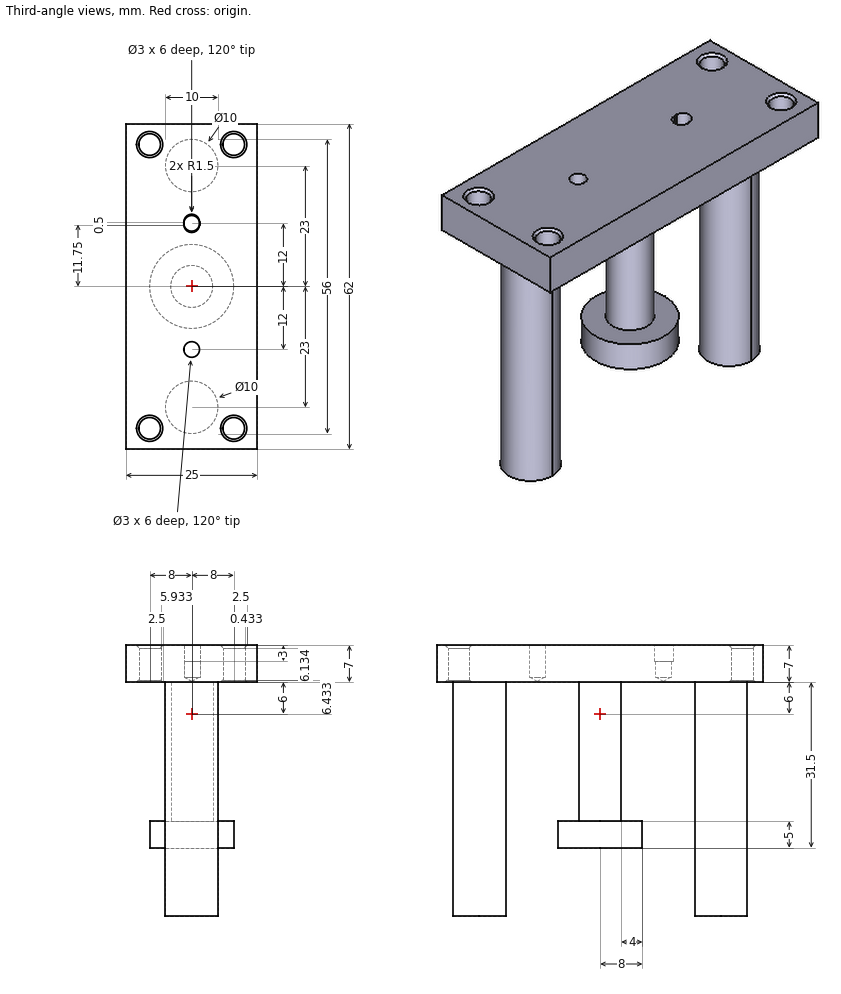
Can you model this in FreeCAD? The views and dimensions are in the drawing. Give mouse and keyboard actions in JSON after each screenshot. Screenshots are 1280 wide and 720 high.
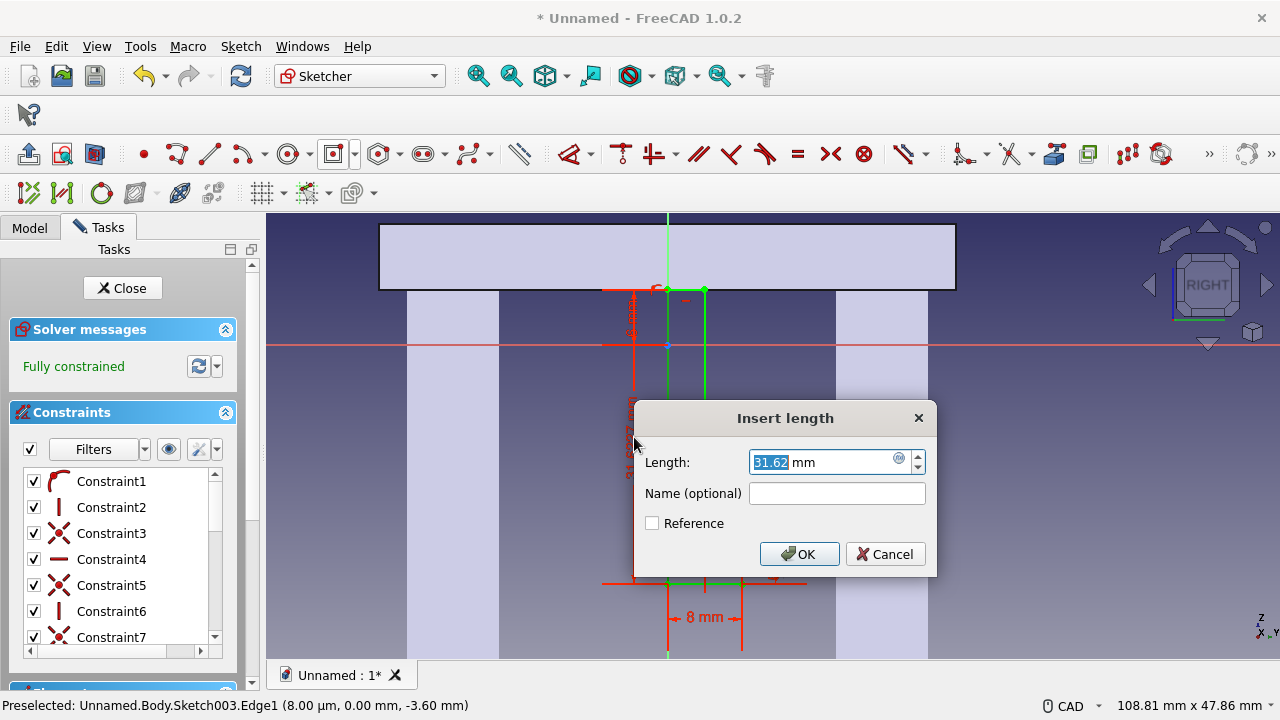
{"action": "type", "text": "31.5"}
{"action": "key", "text": "Return"}
{"action": "key", "text": "Escape"}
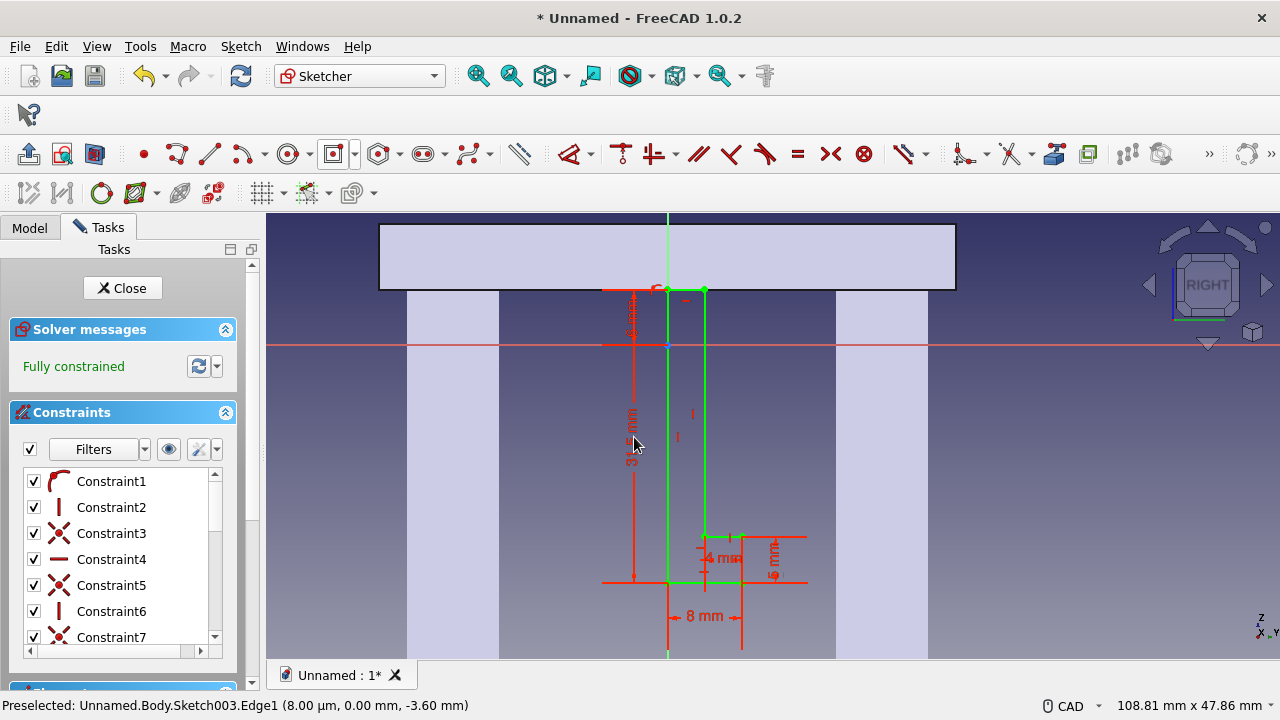
{"action": "left_click", "coordinate": [123, 288]}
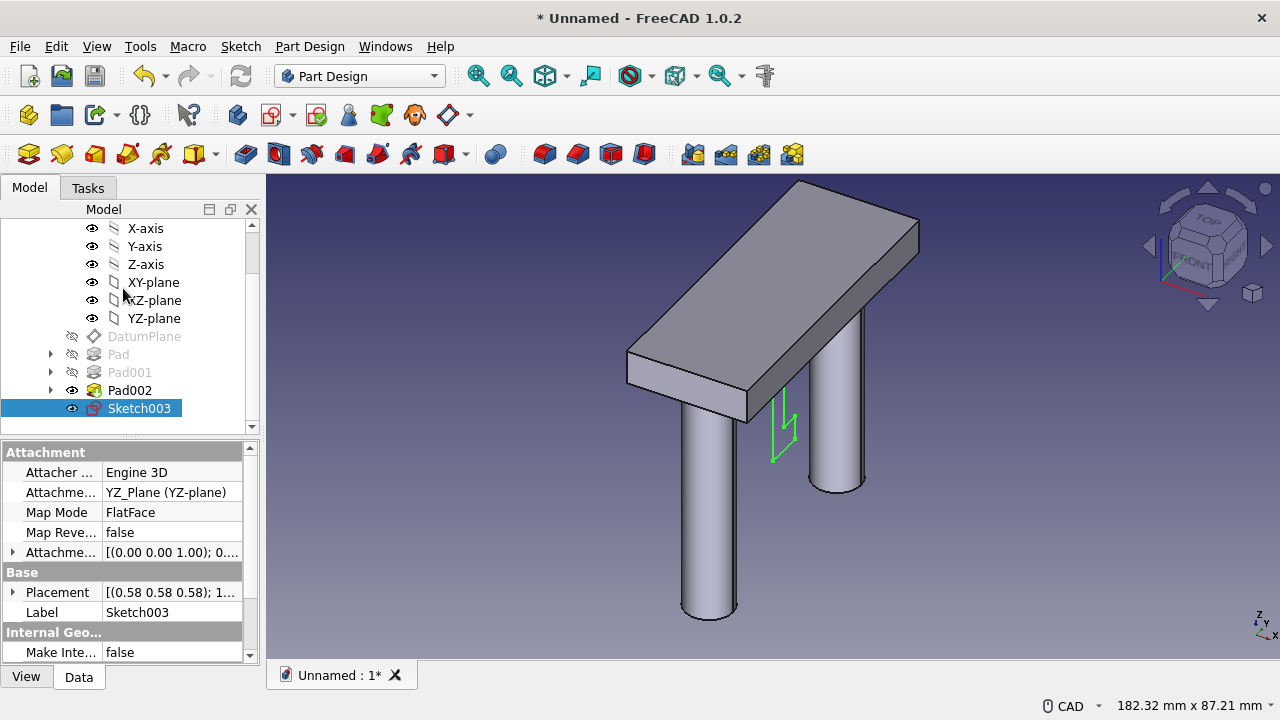
{"action": "left_click", "coordinate": [62, 154]}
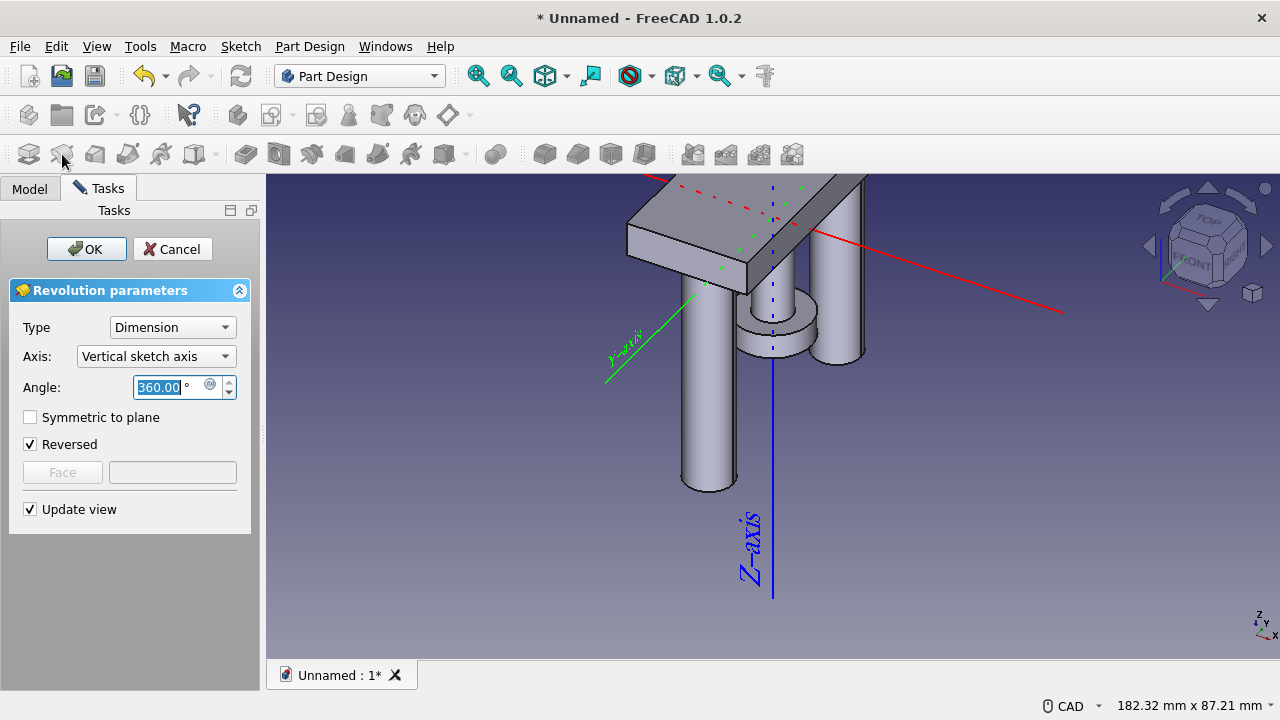
{"action": "left_click", "coordinate": [87, 249]}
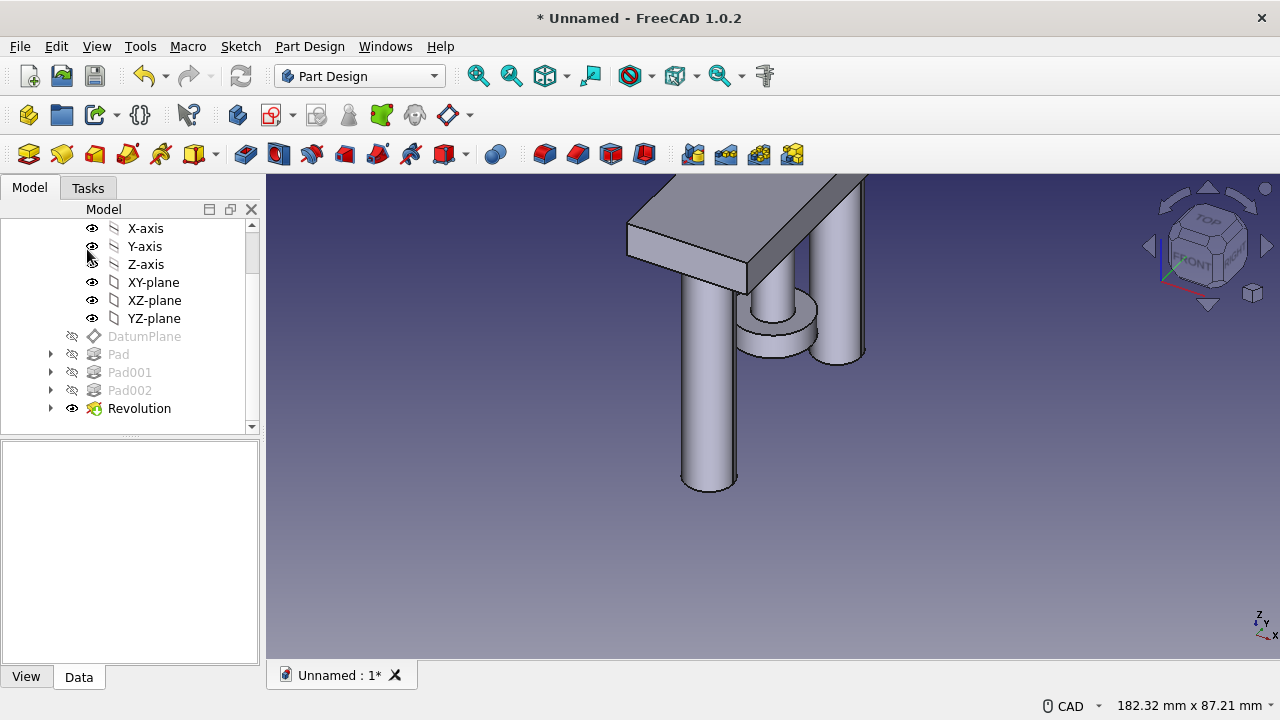
{"action": "left_click", "coordinate": [479, 76]}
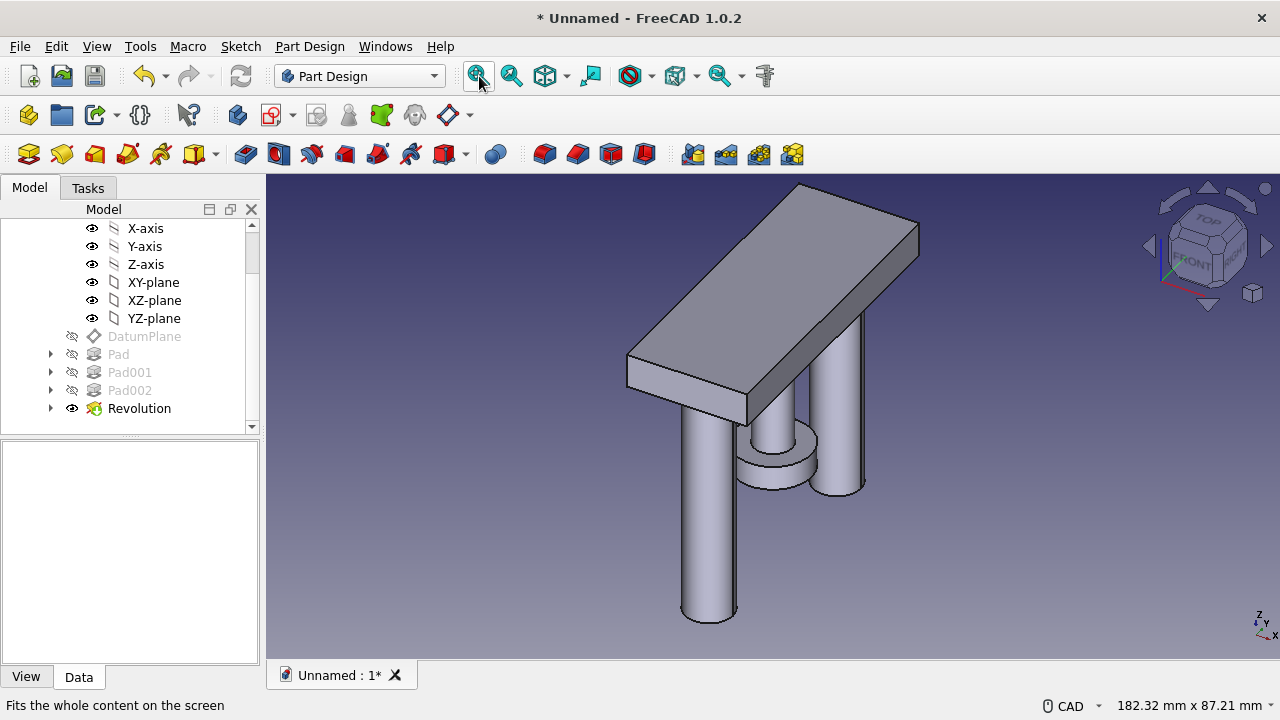
{"action": "left_click", "coordinate": [822, 239]}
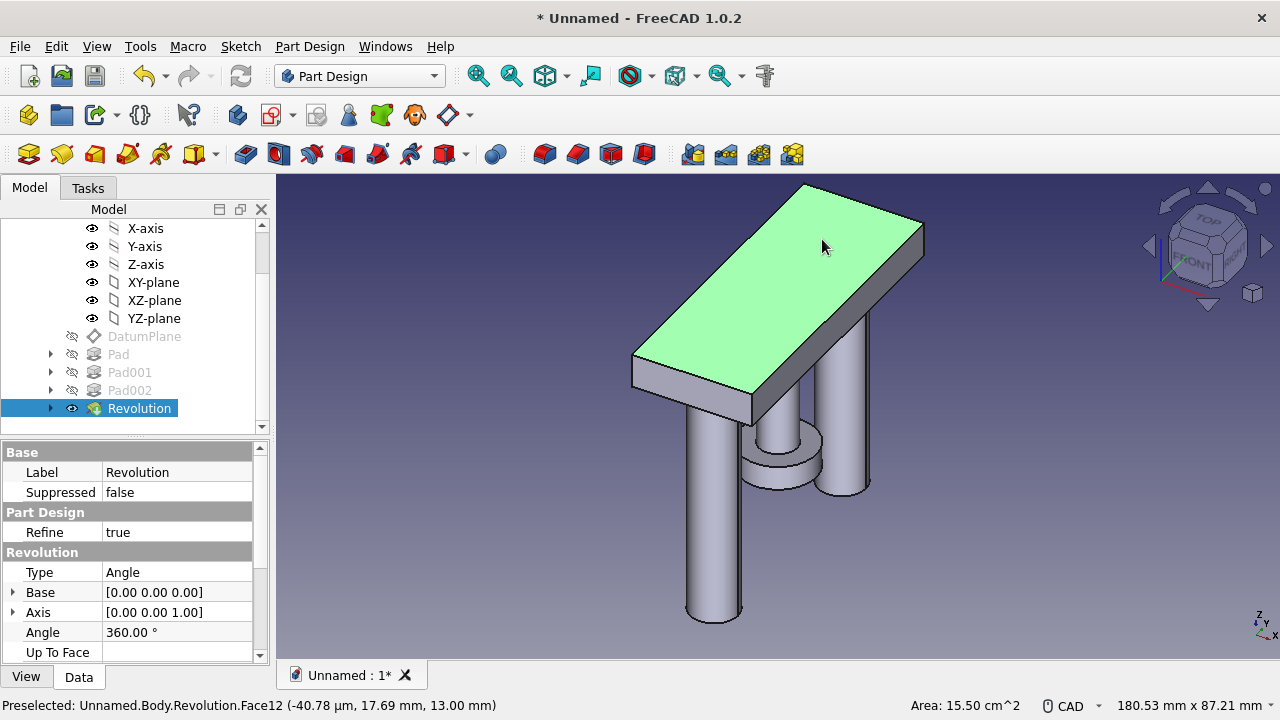
{"action": "left_click", "coordinate": [270, 116]}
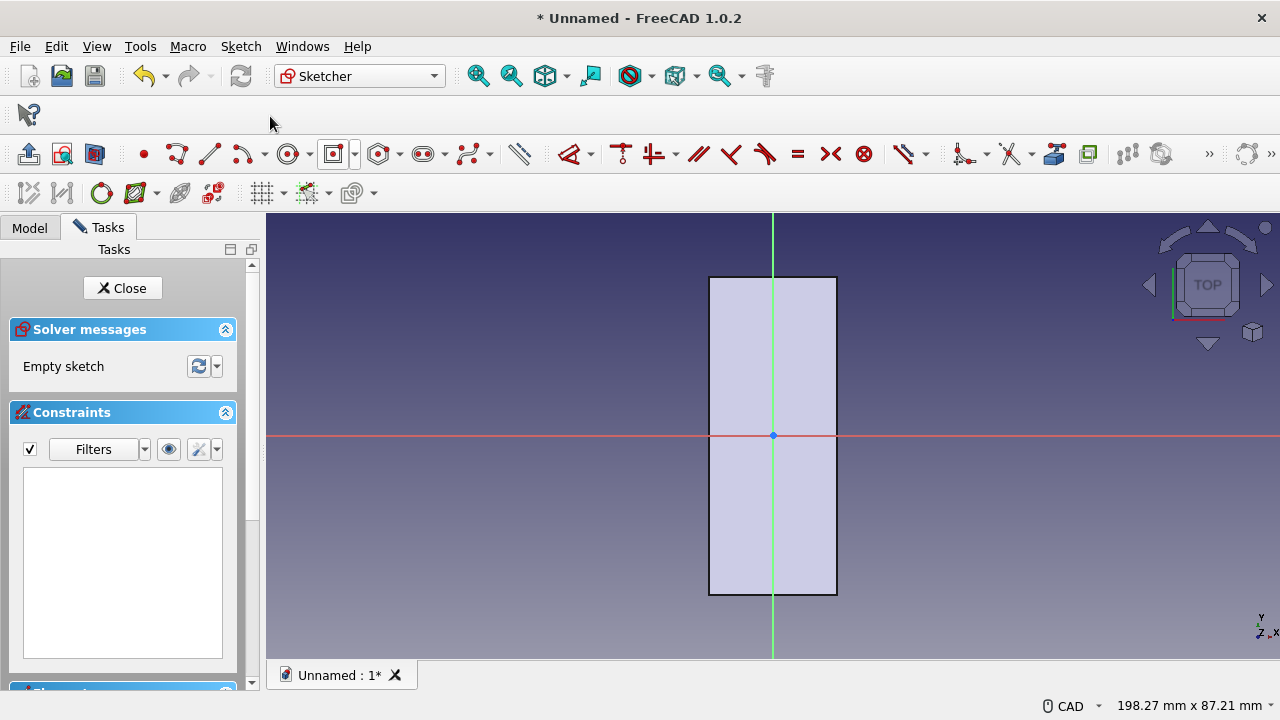
{"action": "scroll", "coordinate": [777, 371], "scroll_direction": "up", "scroll_amount": 14}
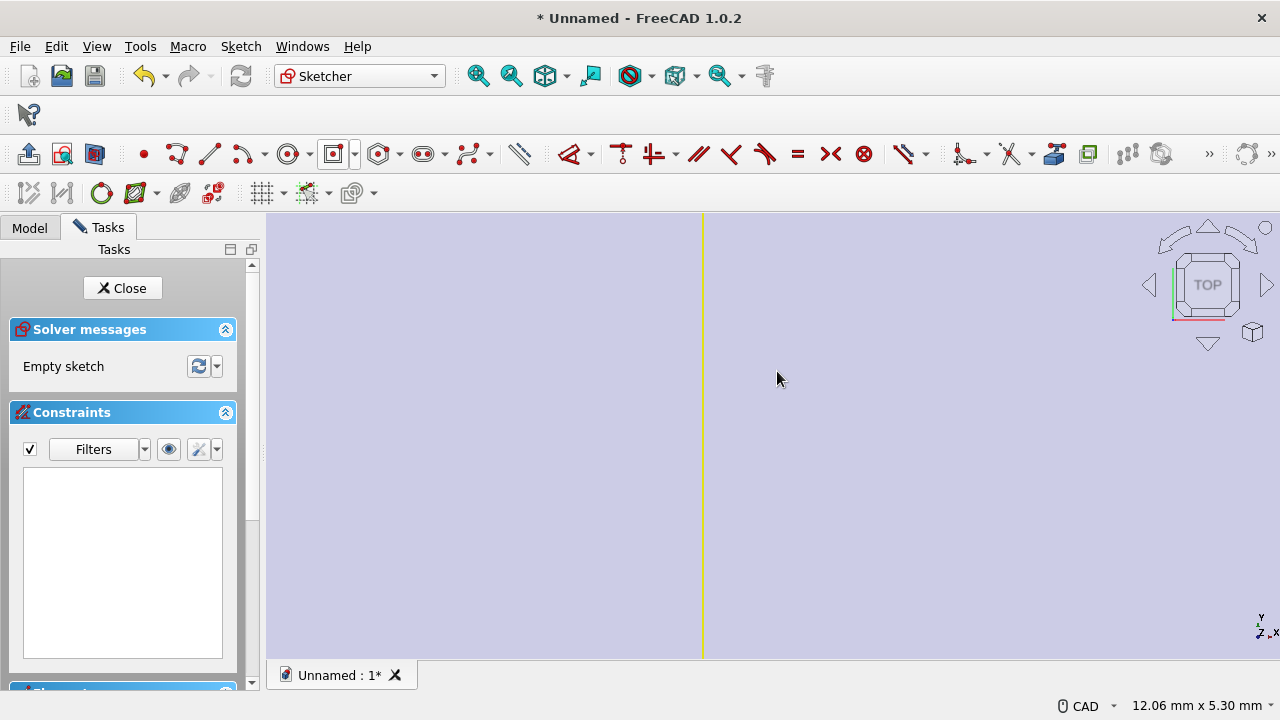
{"action": "left_click", "coordinate": [288, 154]}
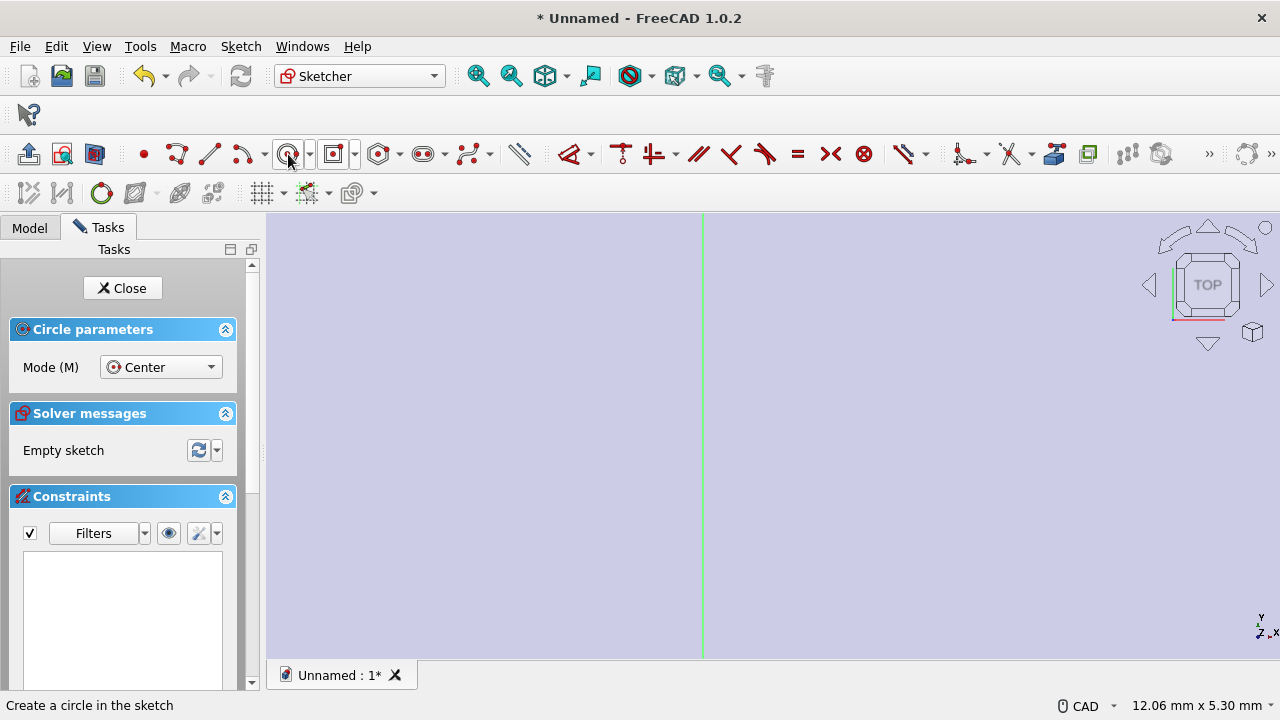
{"action": "left_click", "coordinate": [703, 425]}
{"action": "left_click", "coordinate": [793, 336]}
{"action": "key", "text": "Escape"}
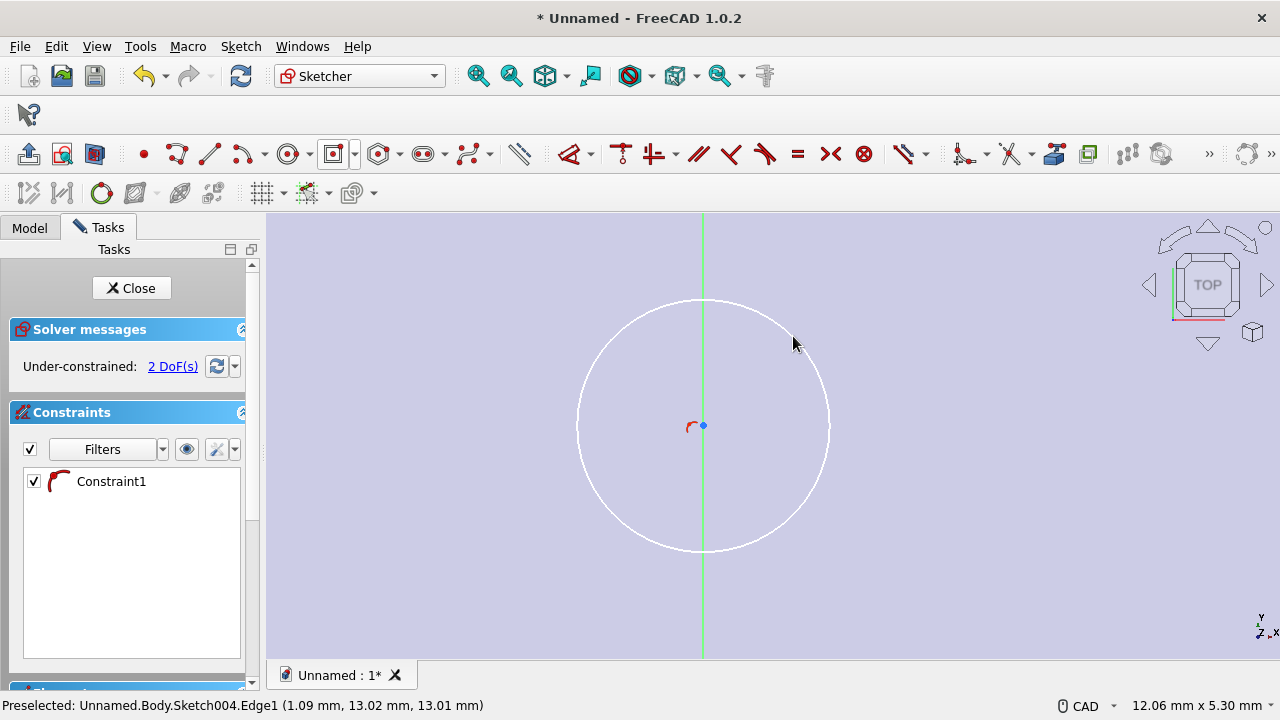
{"action": "left_click", "coordinate": [568, 154]}